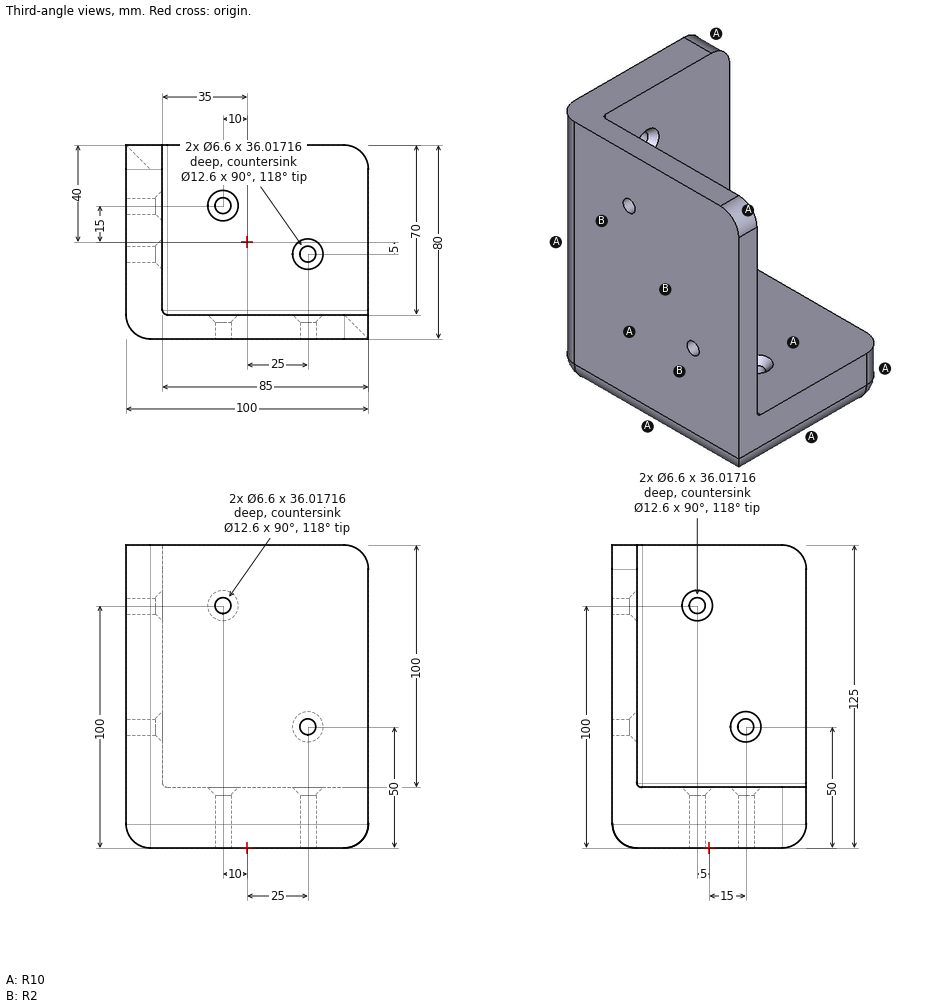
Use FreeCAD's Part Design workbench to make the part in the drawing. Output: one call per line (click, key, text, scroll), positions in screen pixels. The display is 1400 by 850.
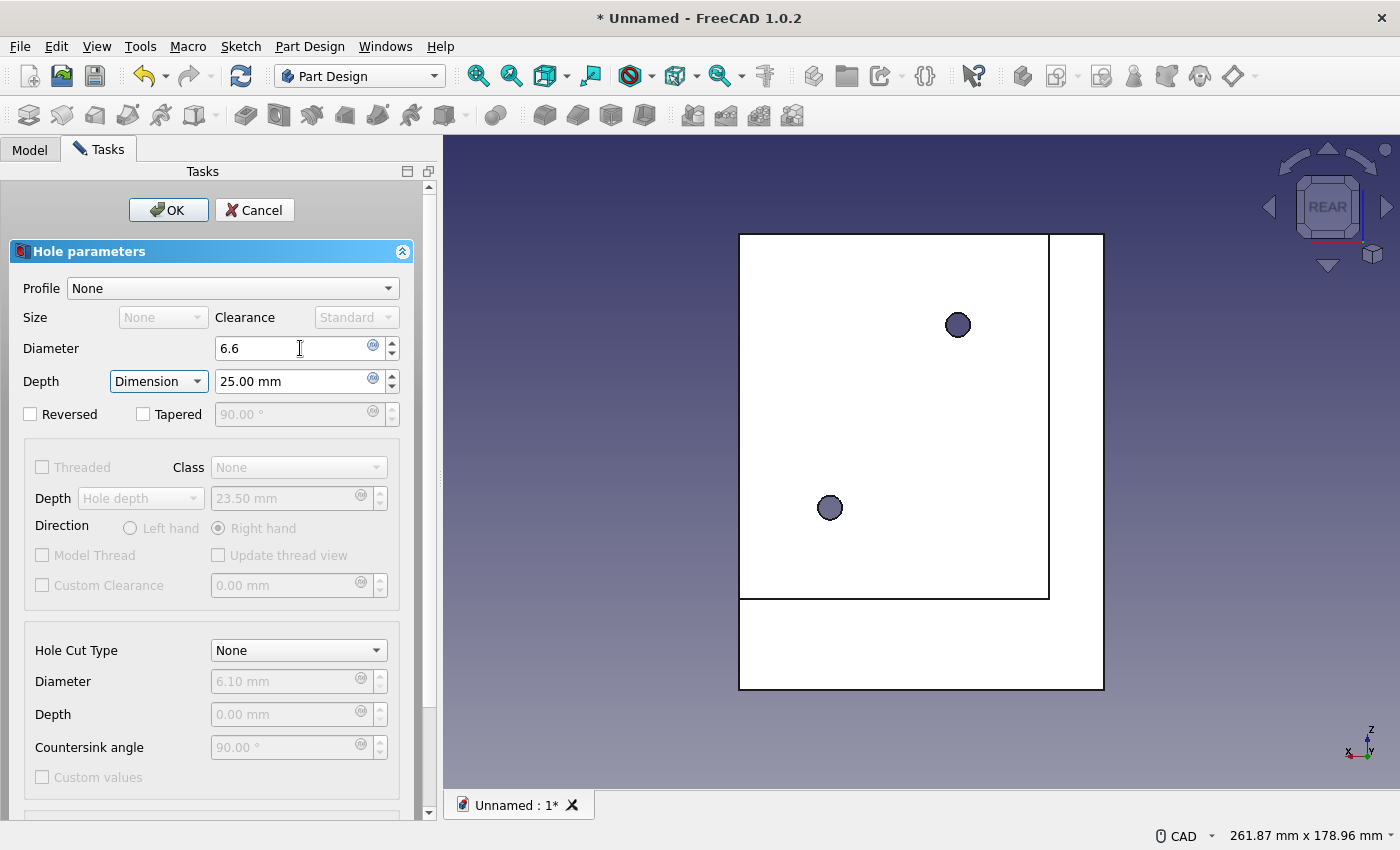
triple_click(300, 382)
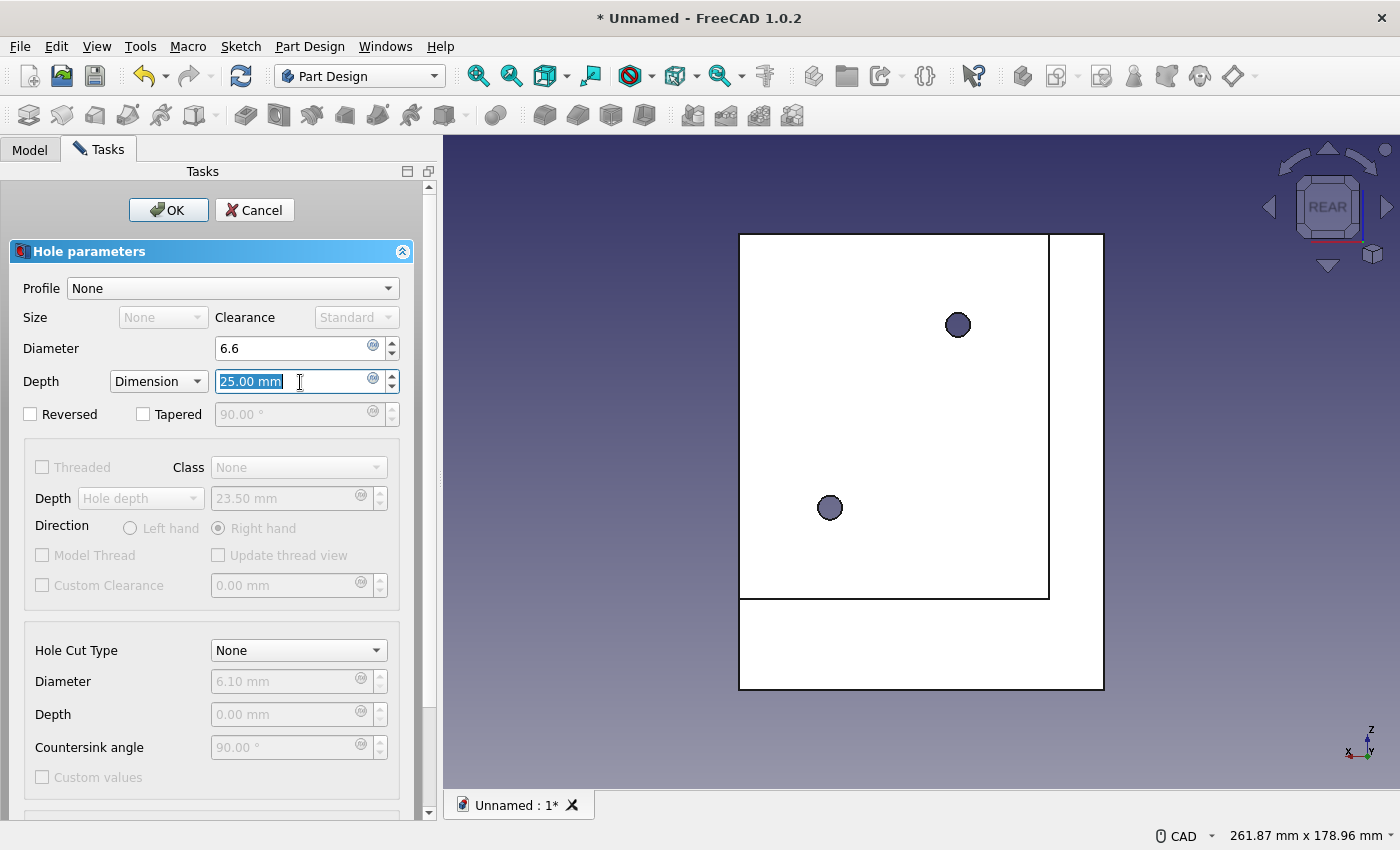
text(36.01716)
key(Tab)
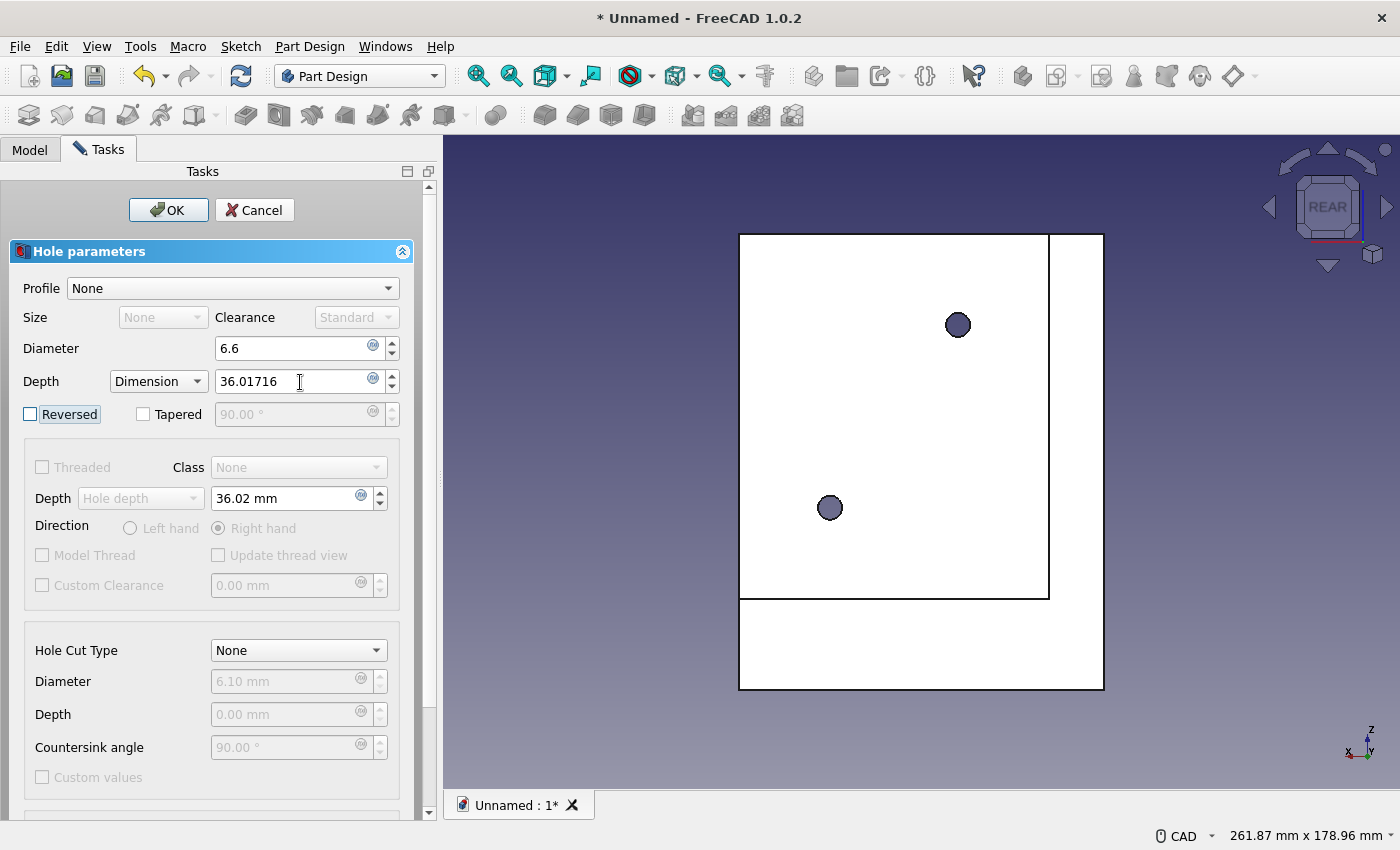
click(300, 650)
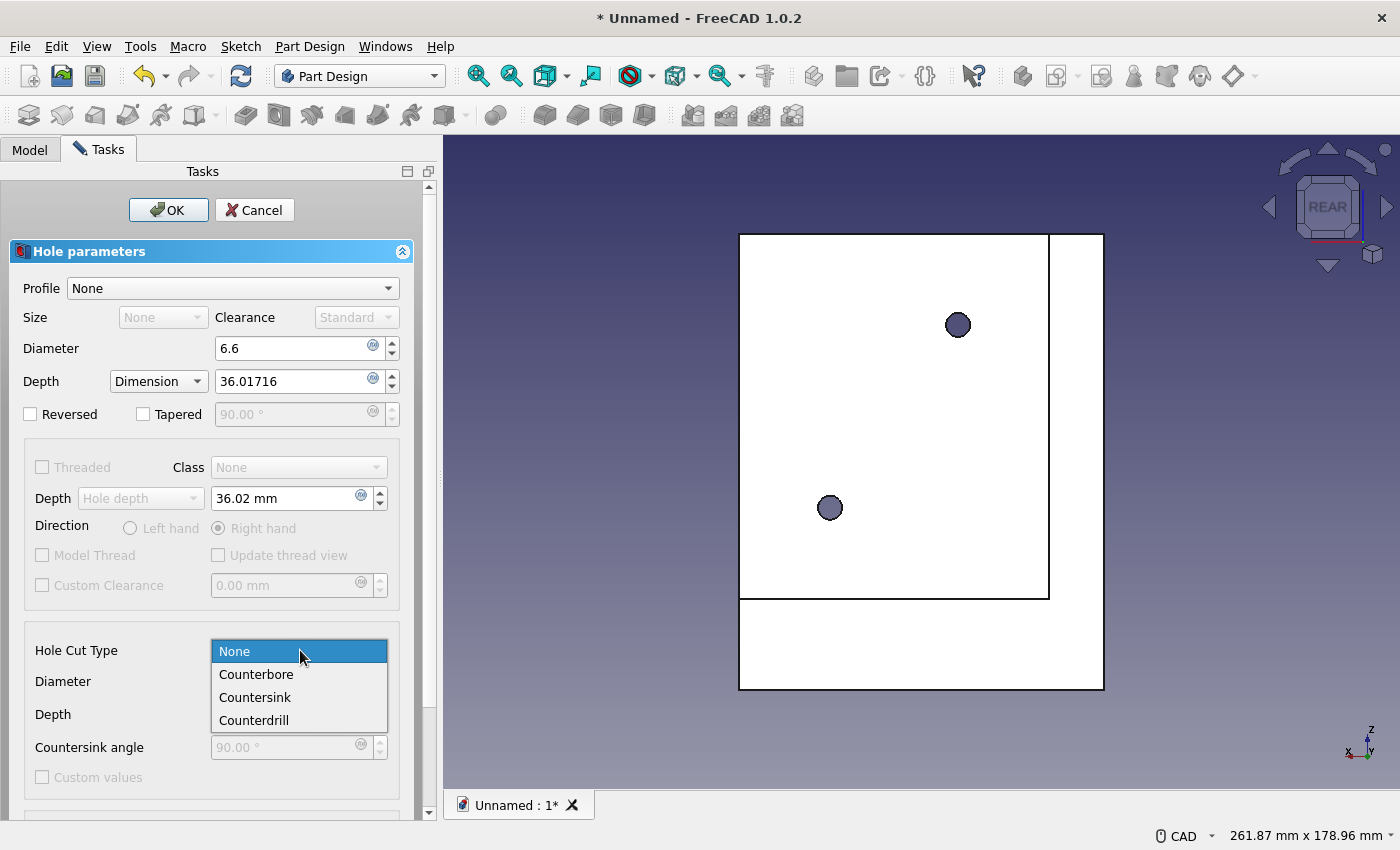
click(298, 698)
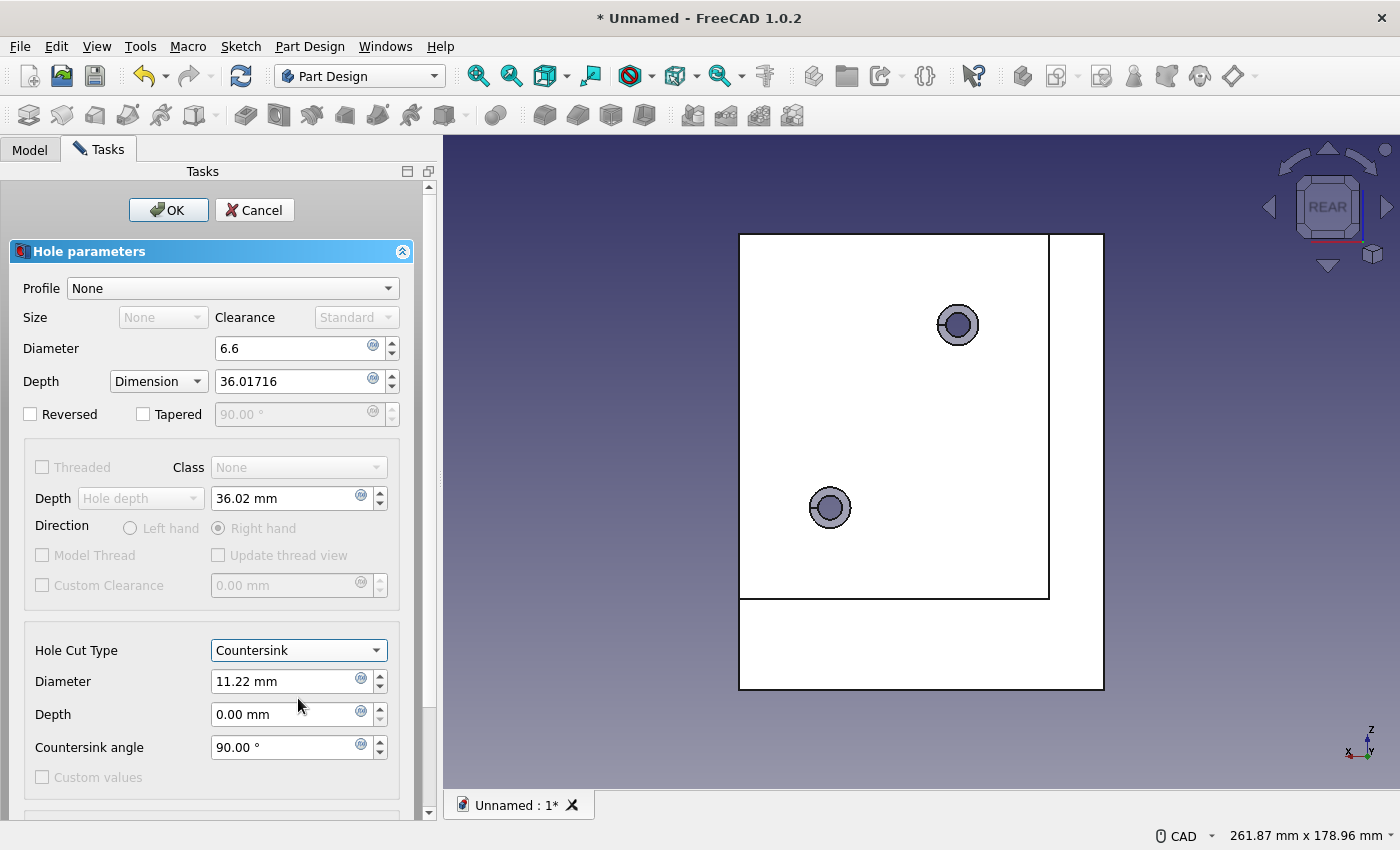
triple_click(292, 682)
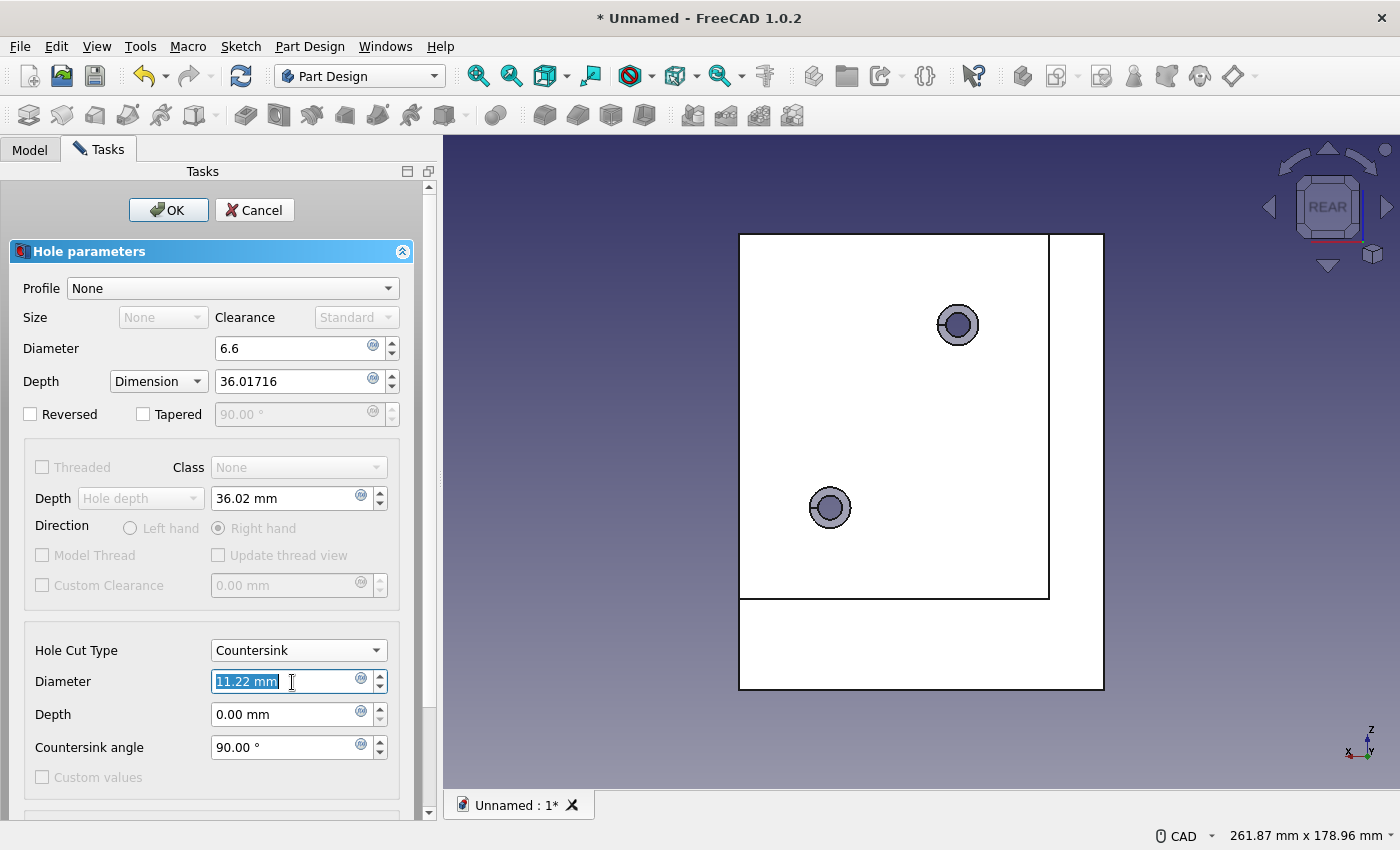
text(12.6)
key(Tab)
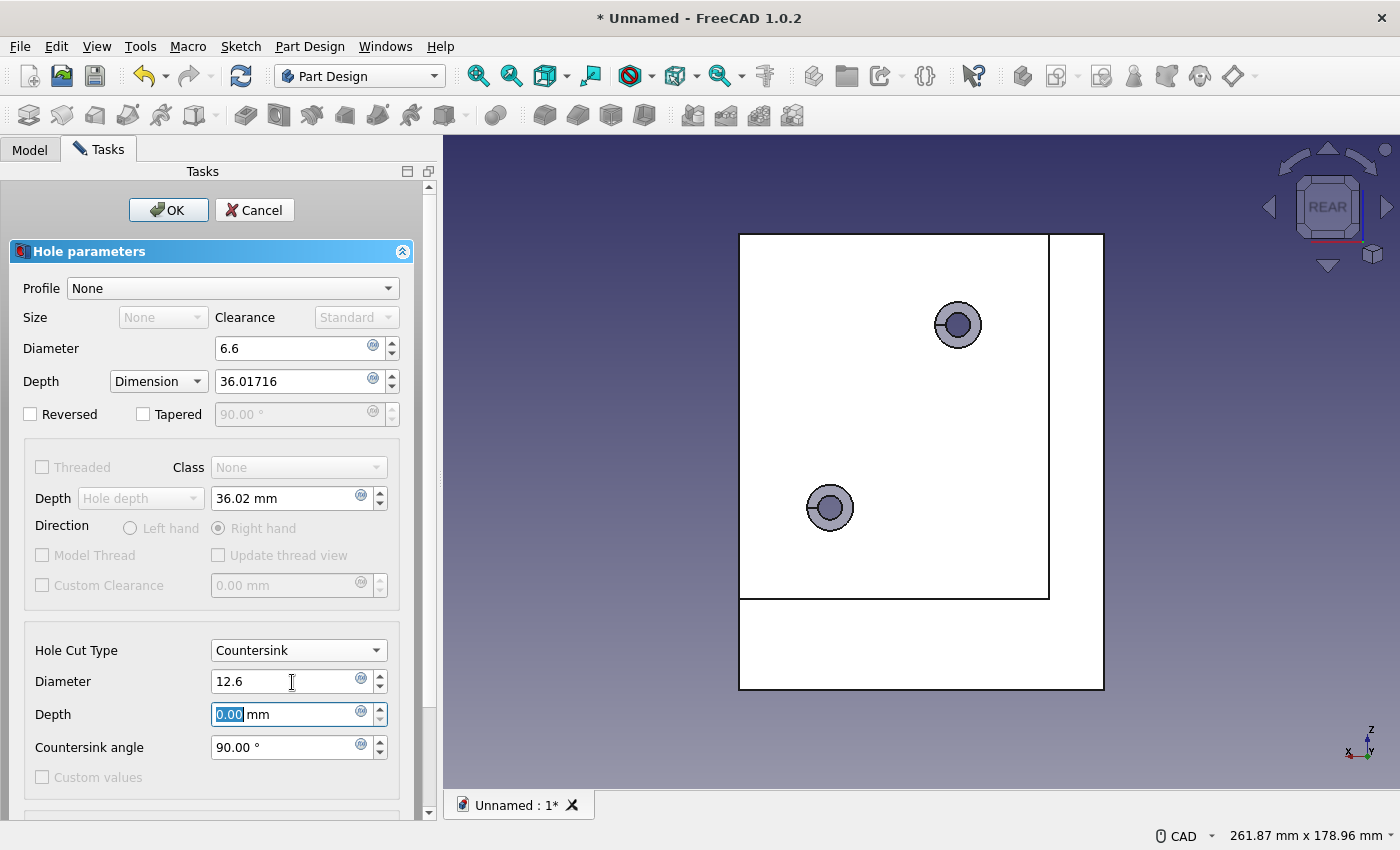
click(169, 210)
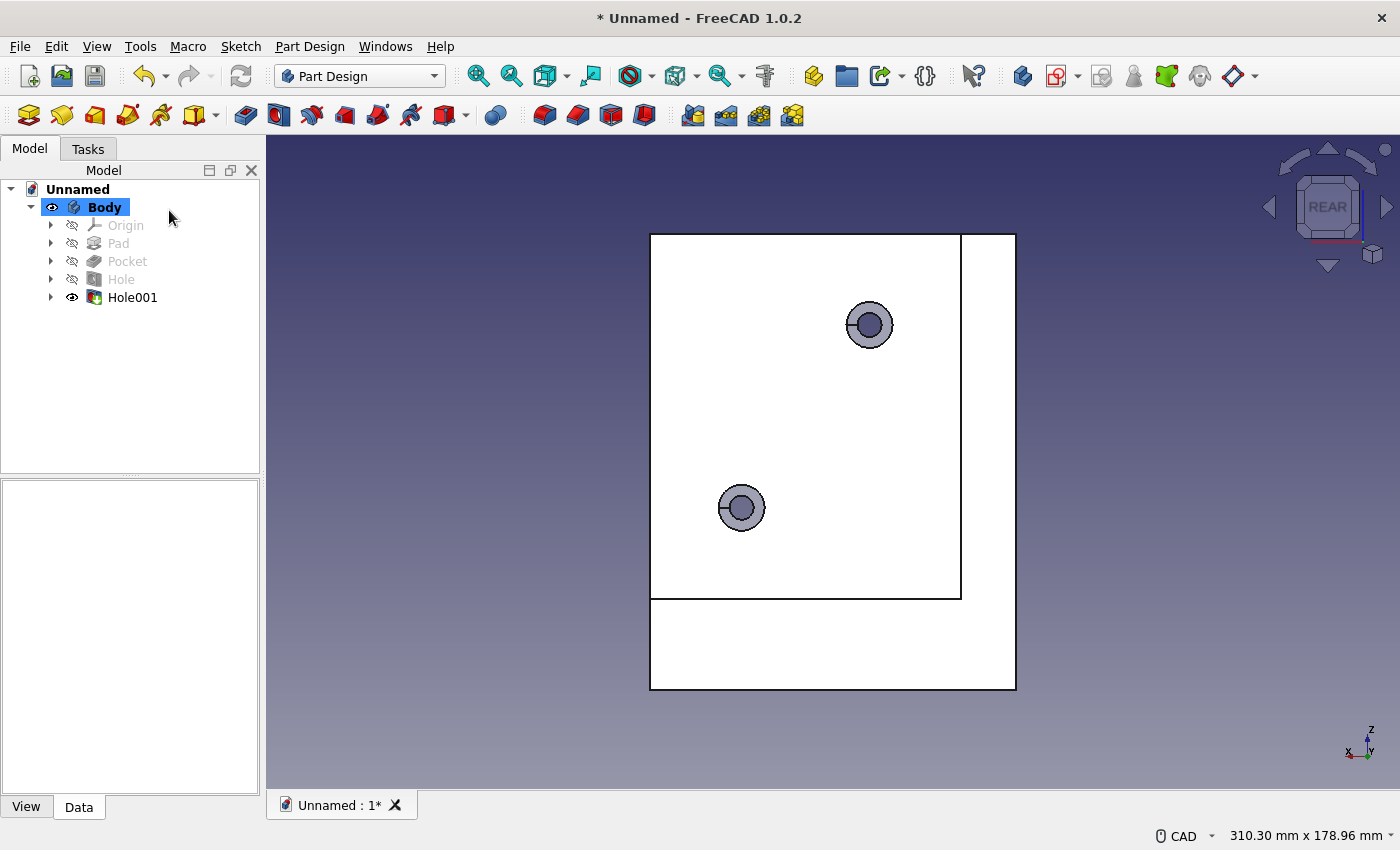
key(0)